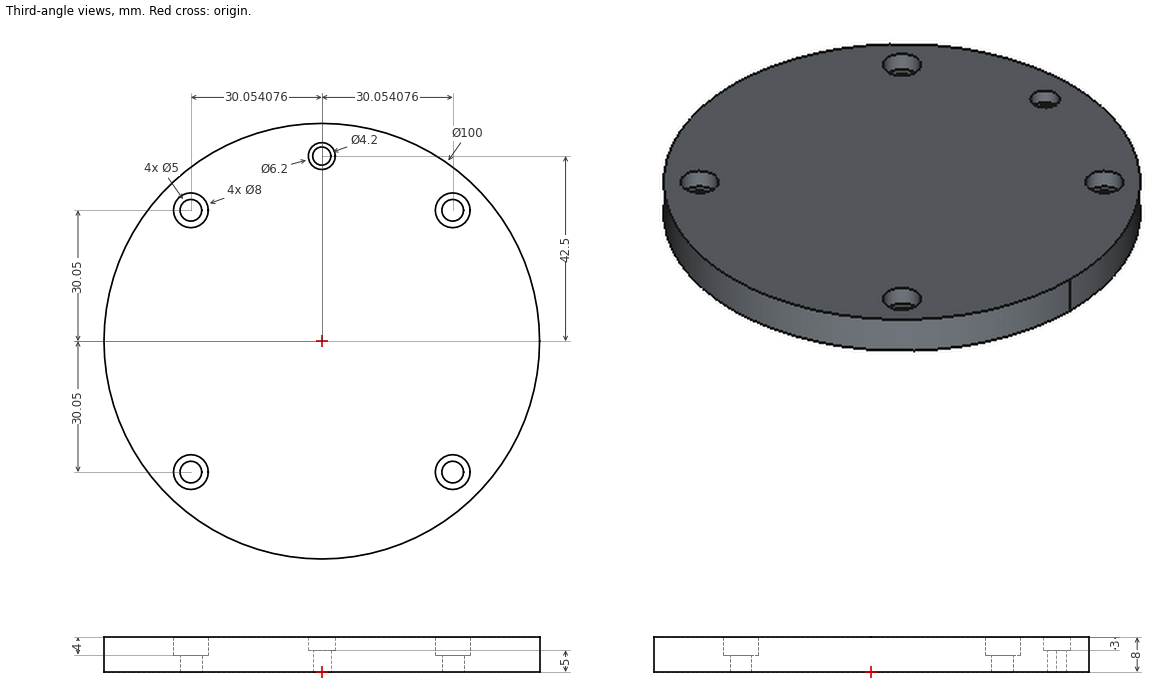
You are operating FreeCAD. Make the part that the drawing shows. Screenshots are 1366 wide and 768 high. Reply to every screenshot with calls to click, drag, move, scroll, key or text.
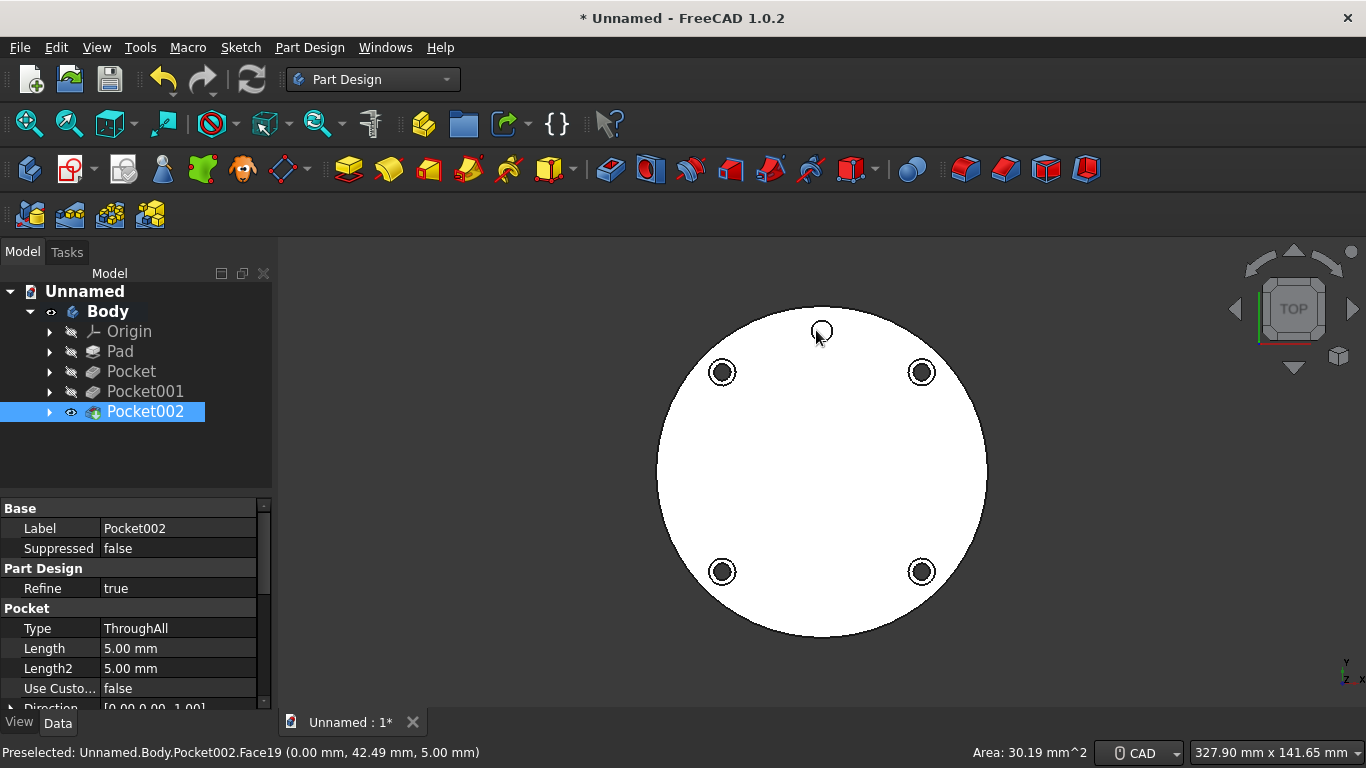
click(70, 170)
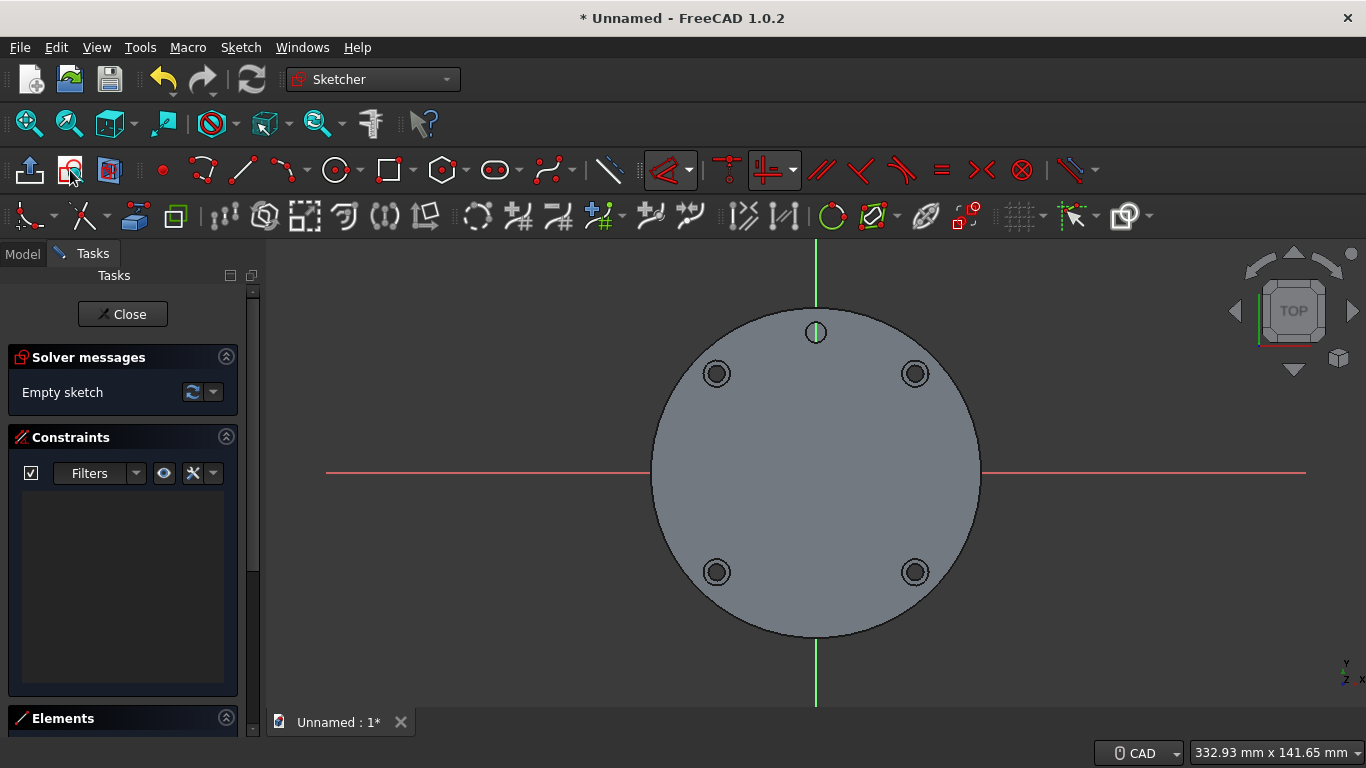
scroll(820, 325, up, 15)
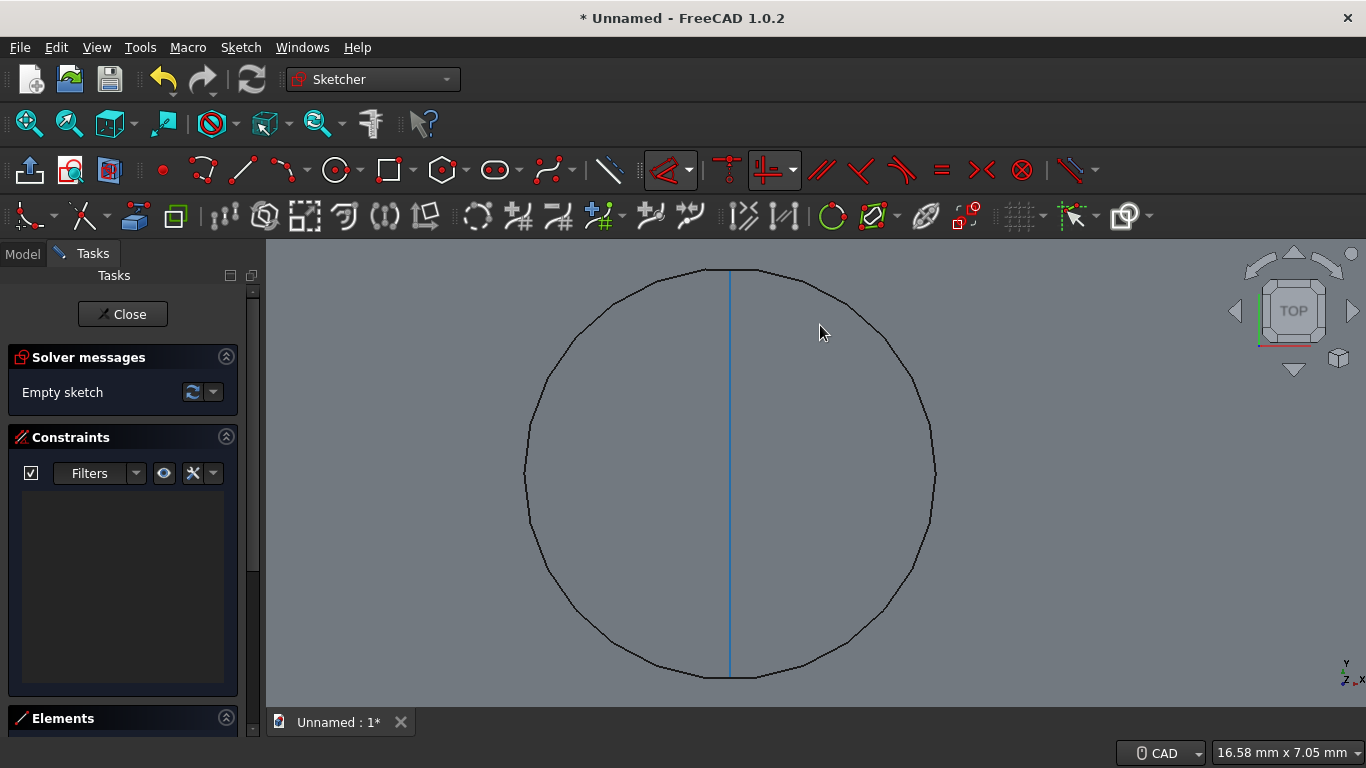
key(g)
key(c)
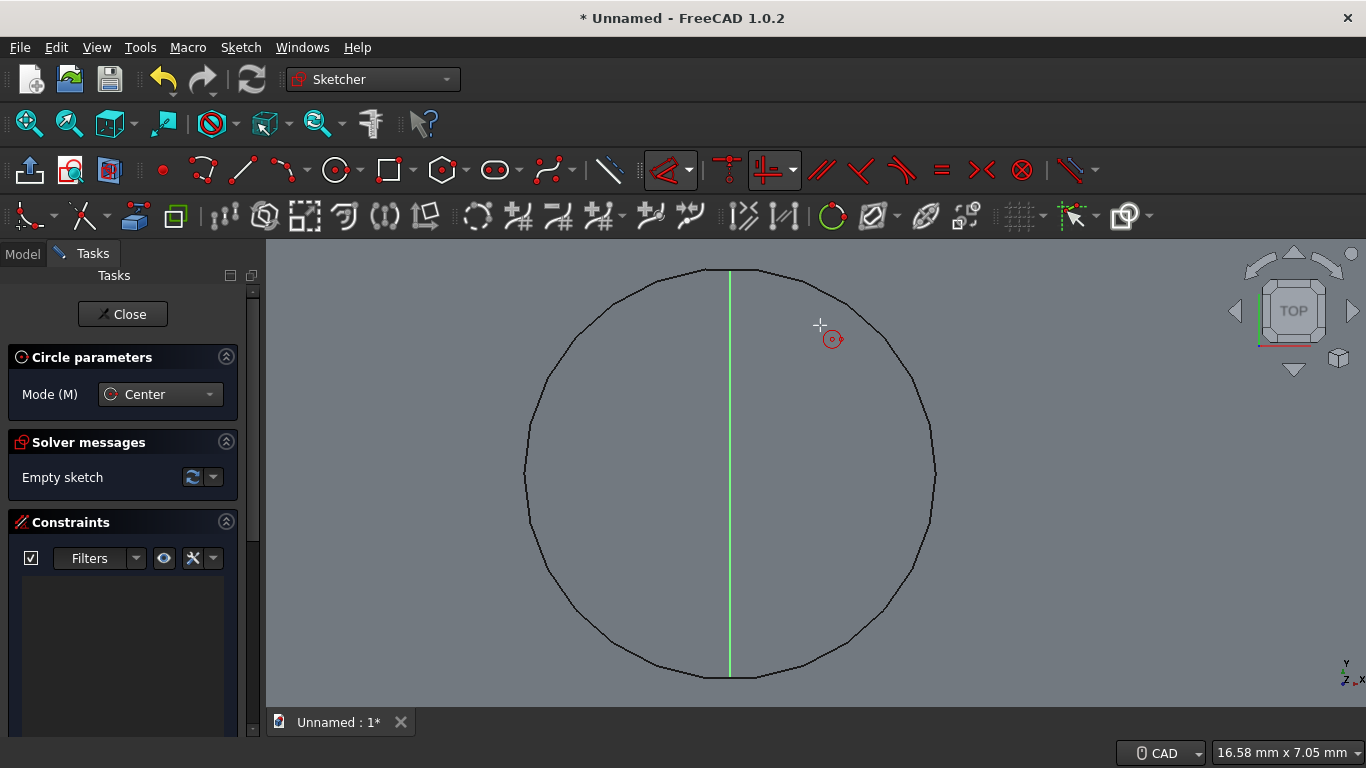
click(730, 474)
move(829, 375)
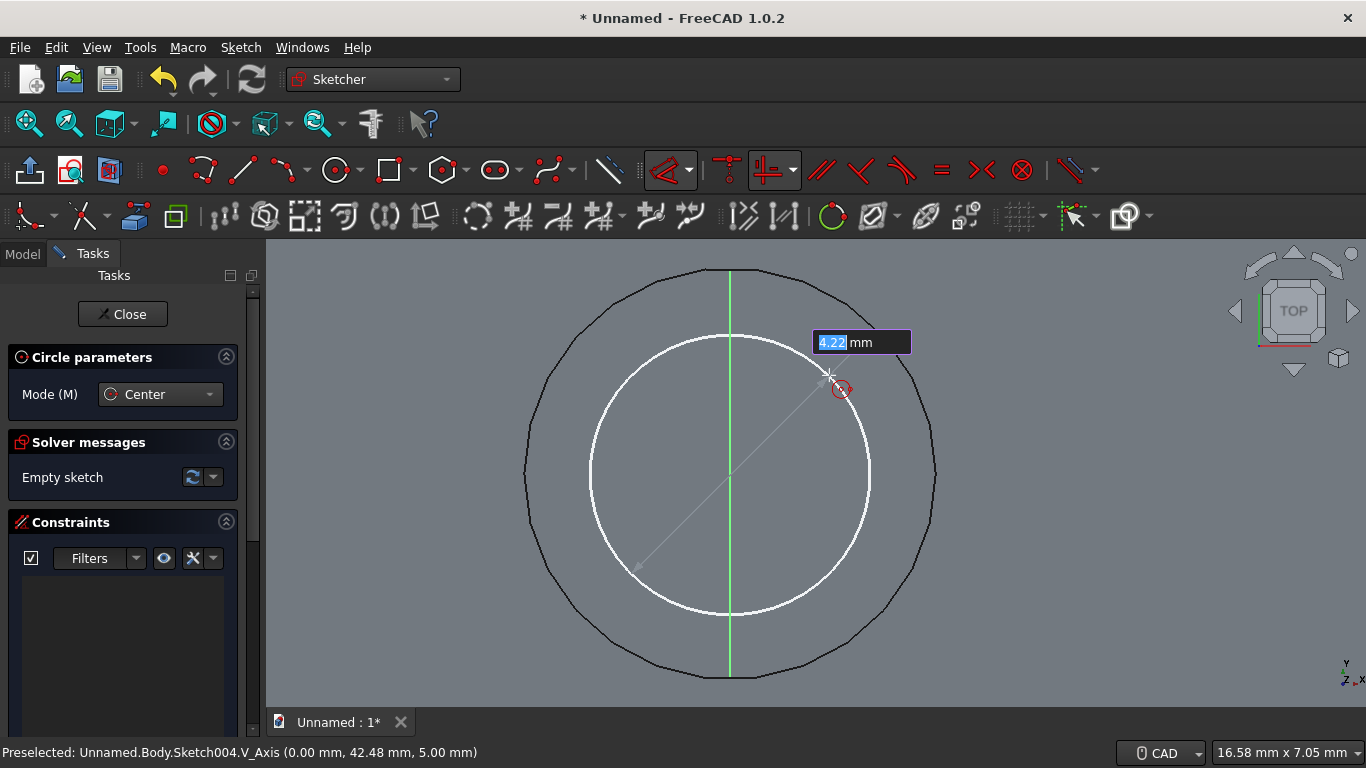
text(4.2)
key(Return)
key(Escape)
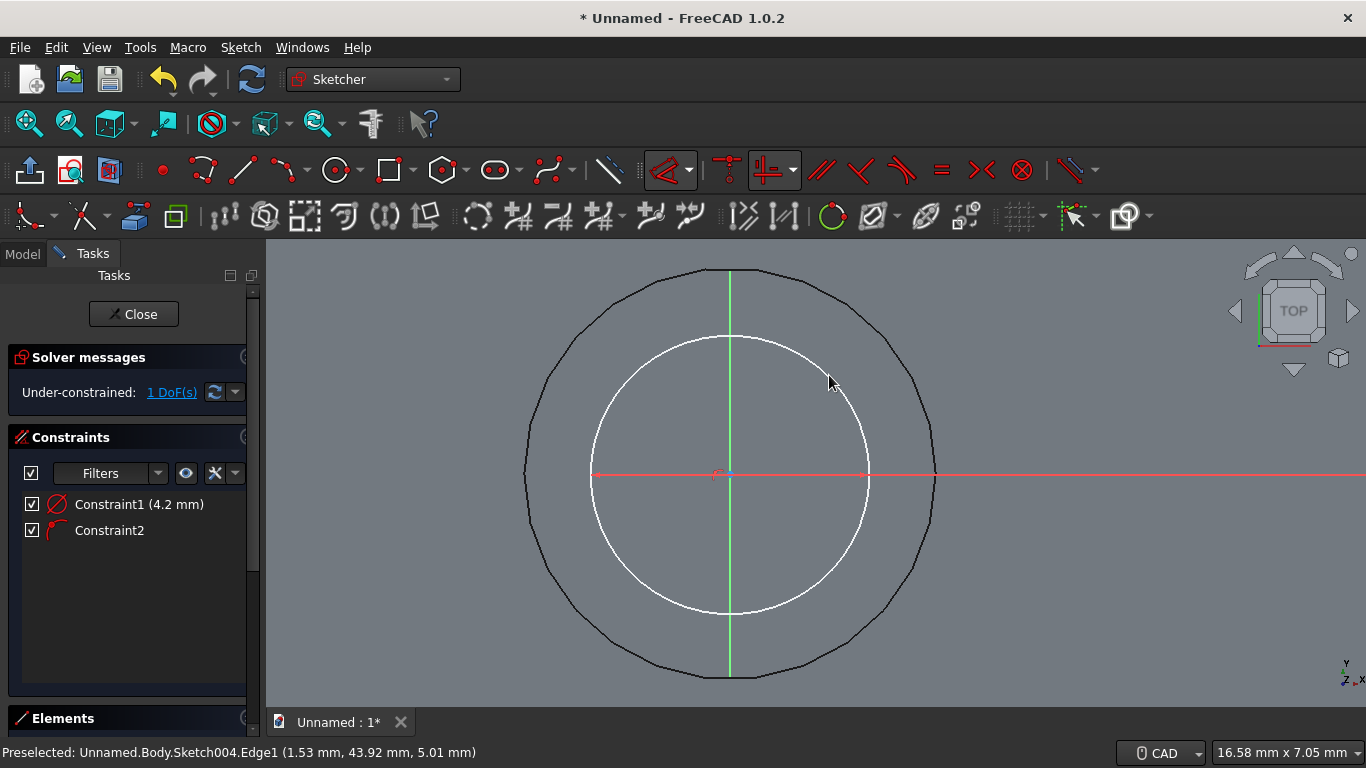
click(730, 475)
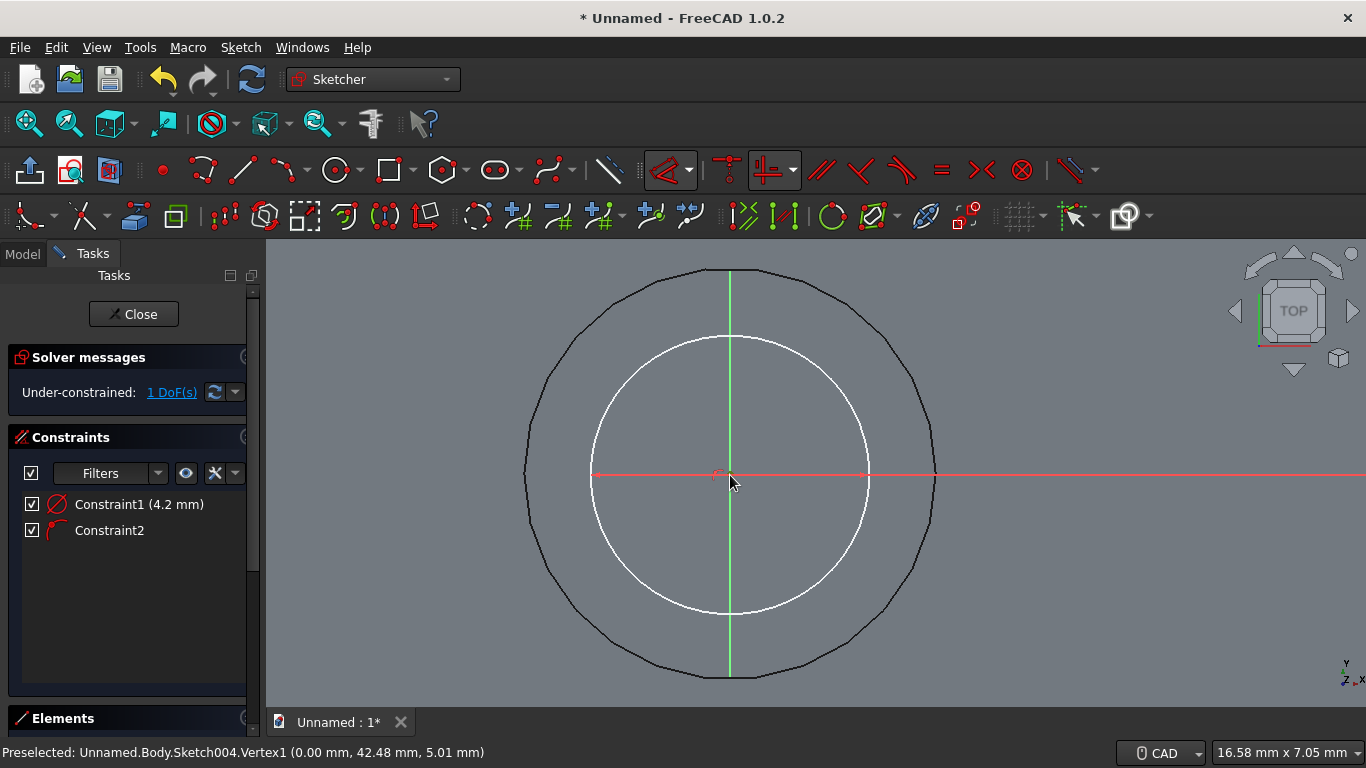
key(i)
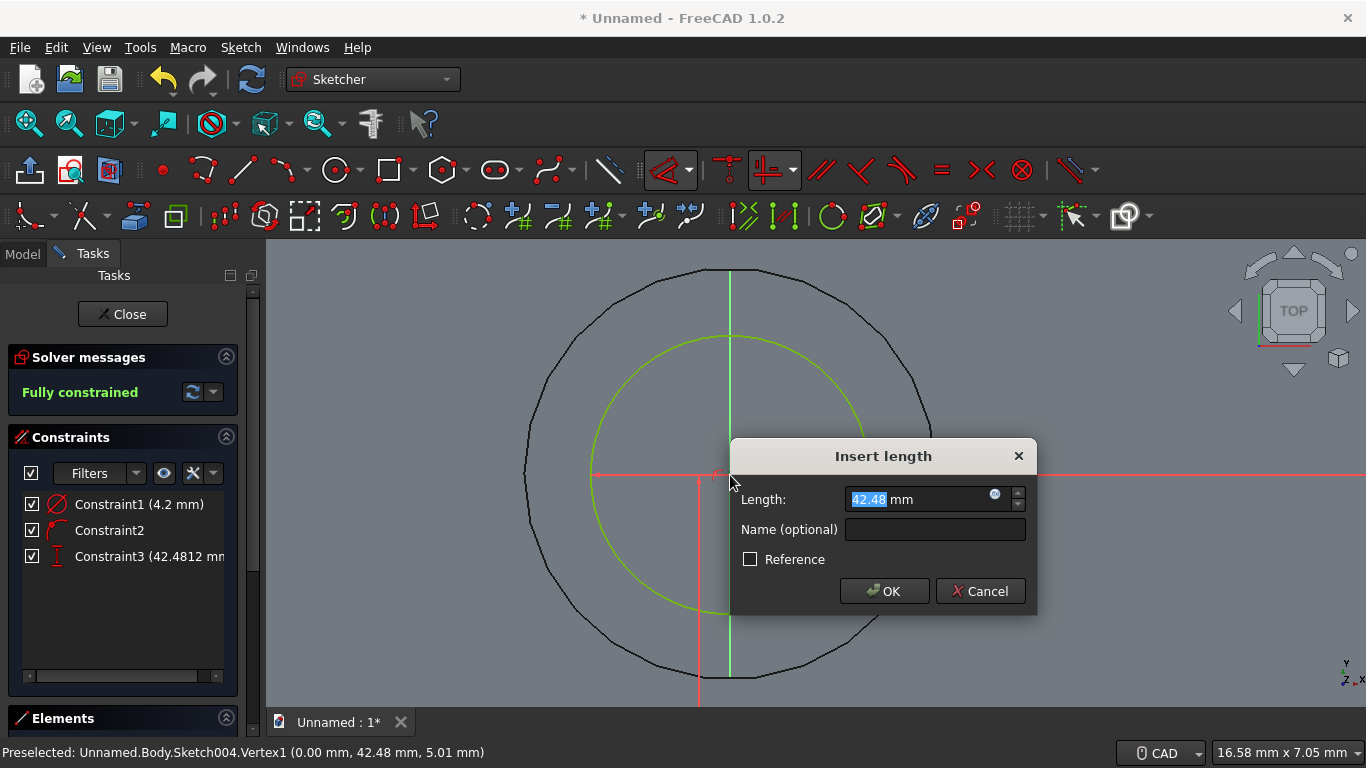
text(42.5)
key(Return)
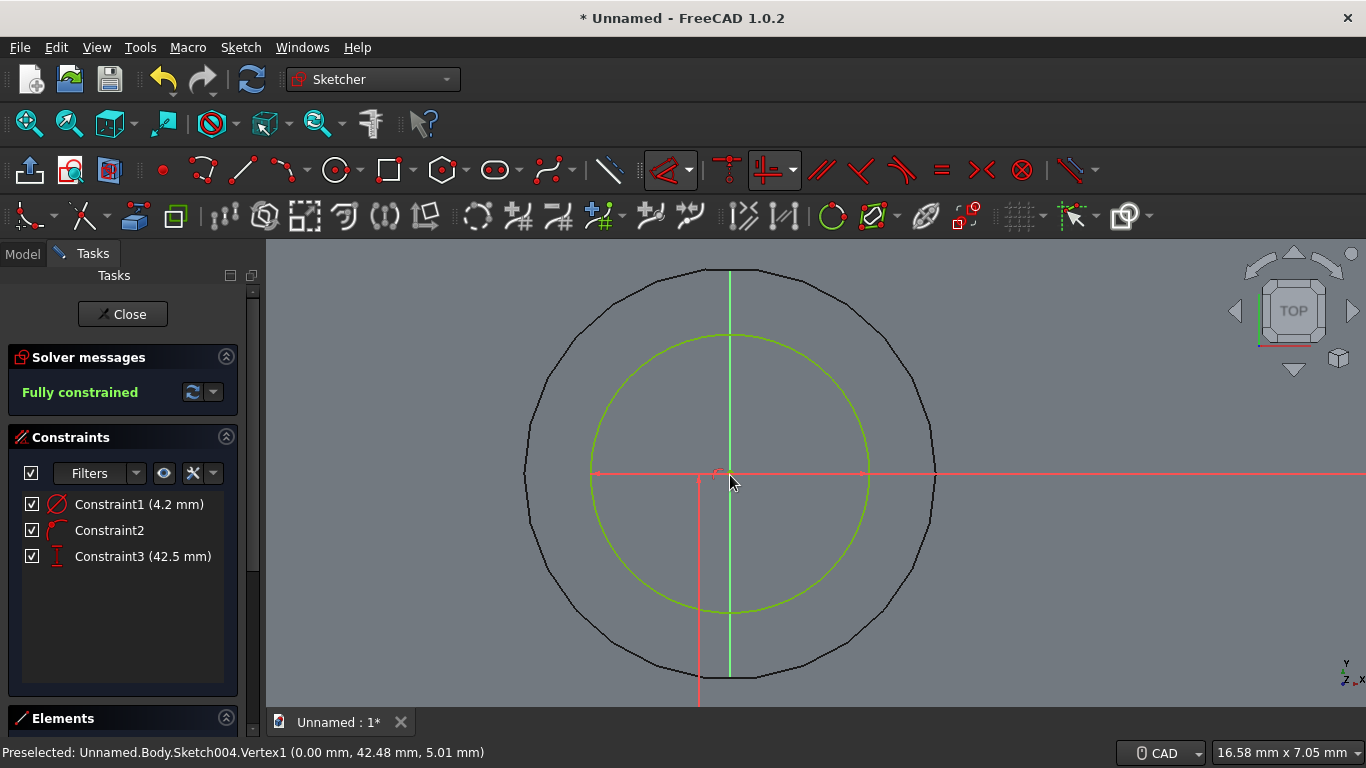
click(123, 314)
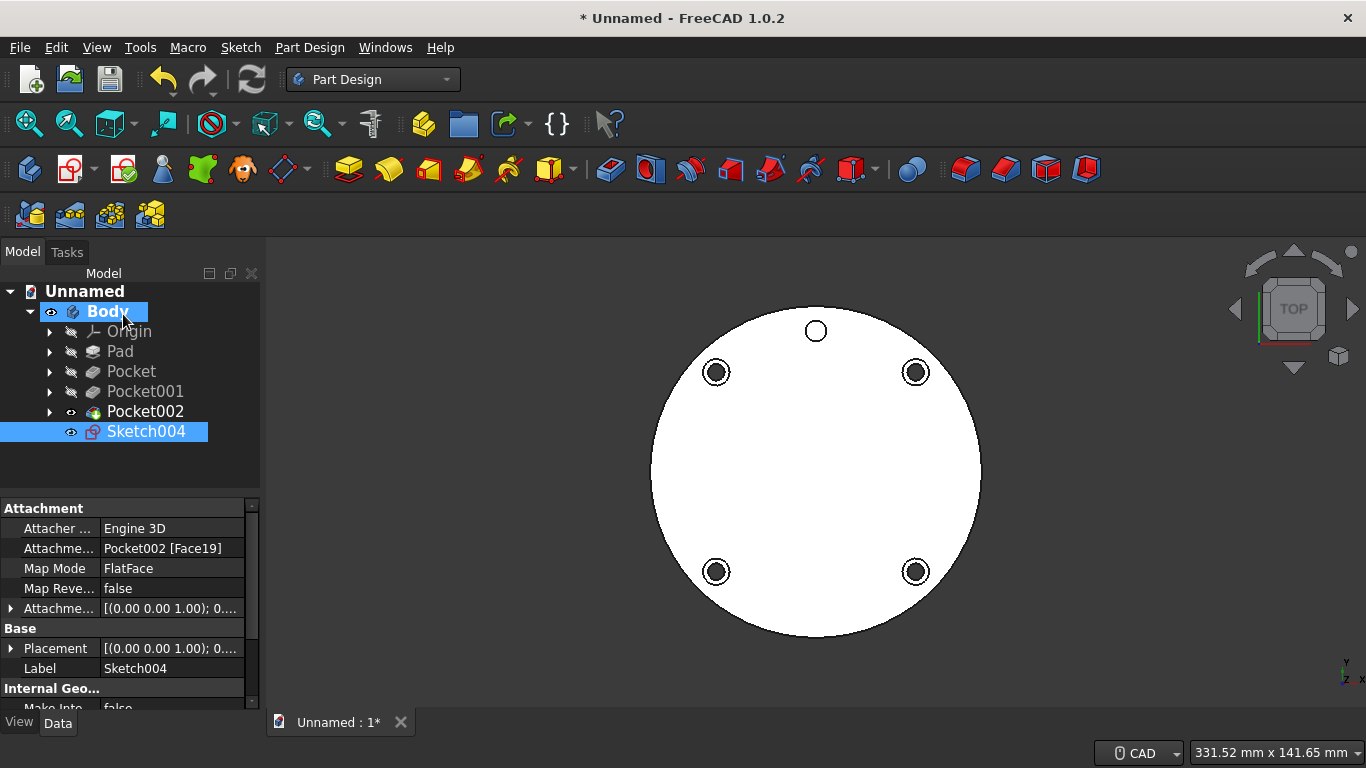
click(612, 170)